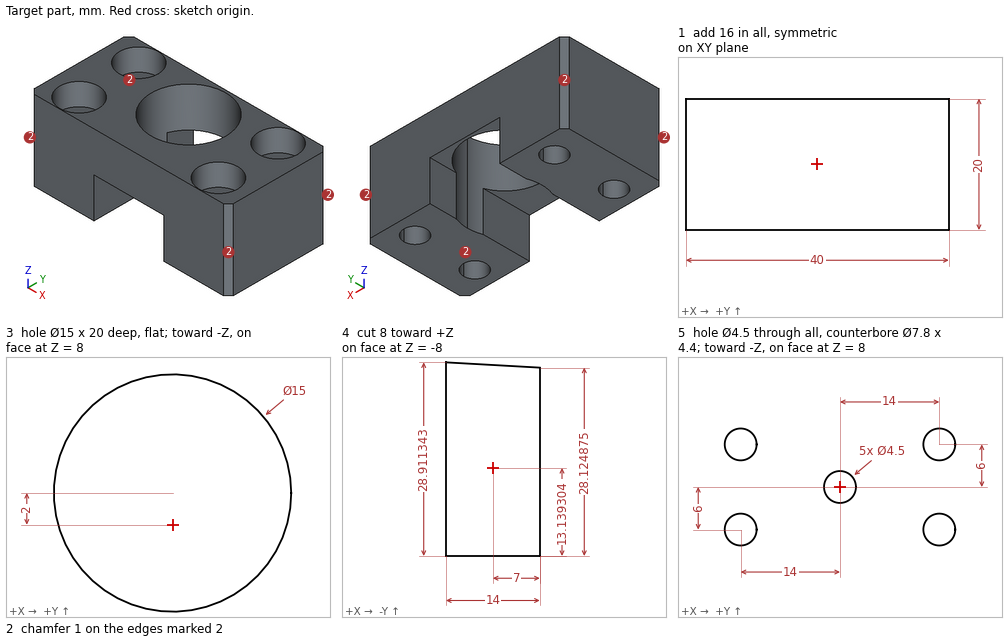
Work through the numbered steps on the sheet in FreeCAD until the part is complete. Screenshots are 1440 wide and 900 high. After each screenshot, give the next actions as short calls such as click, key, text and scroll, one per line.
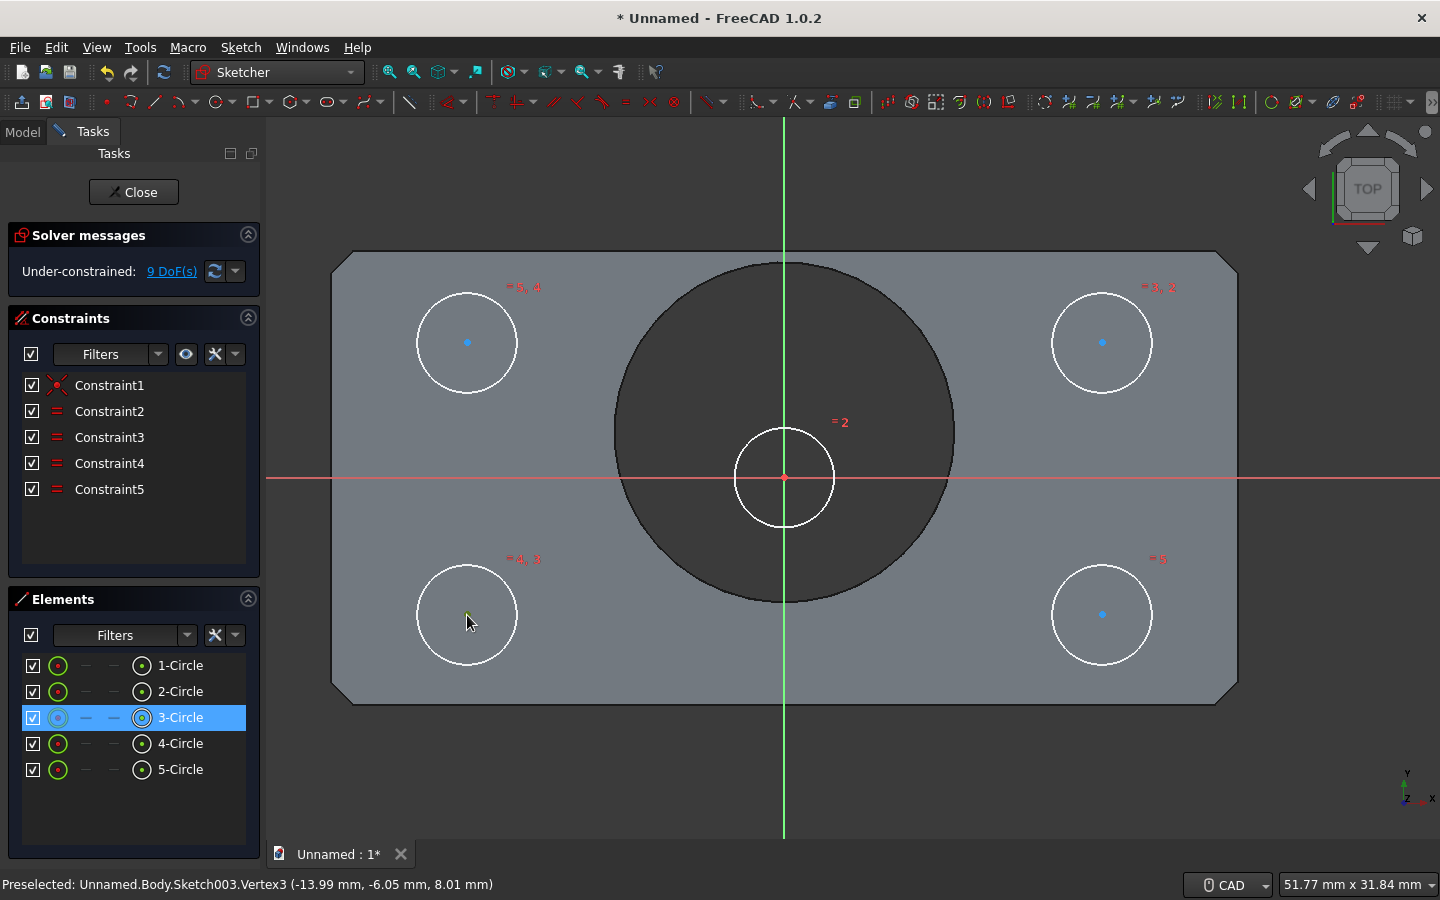
click(467, 343)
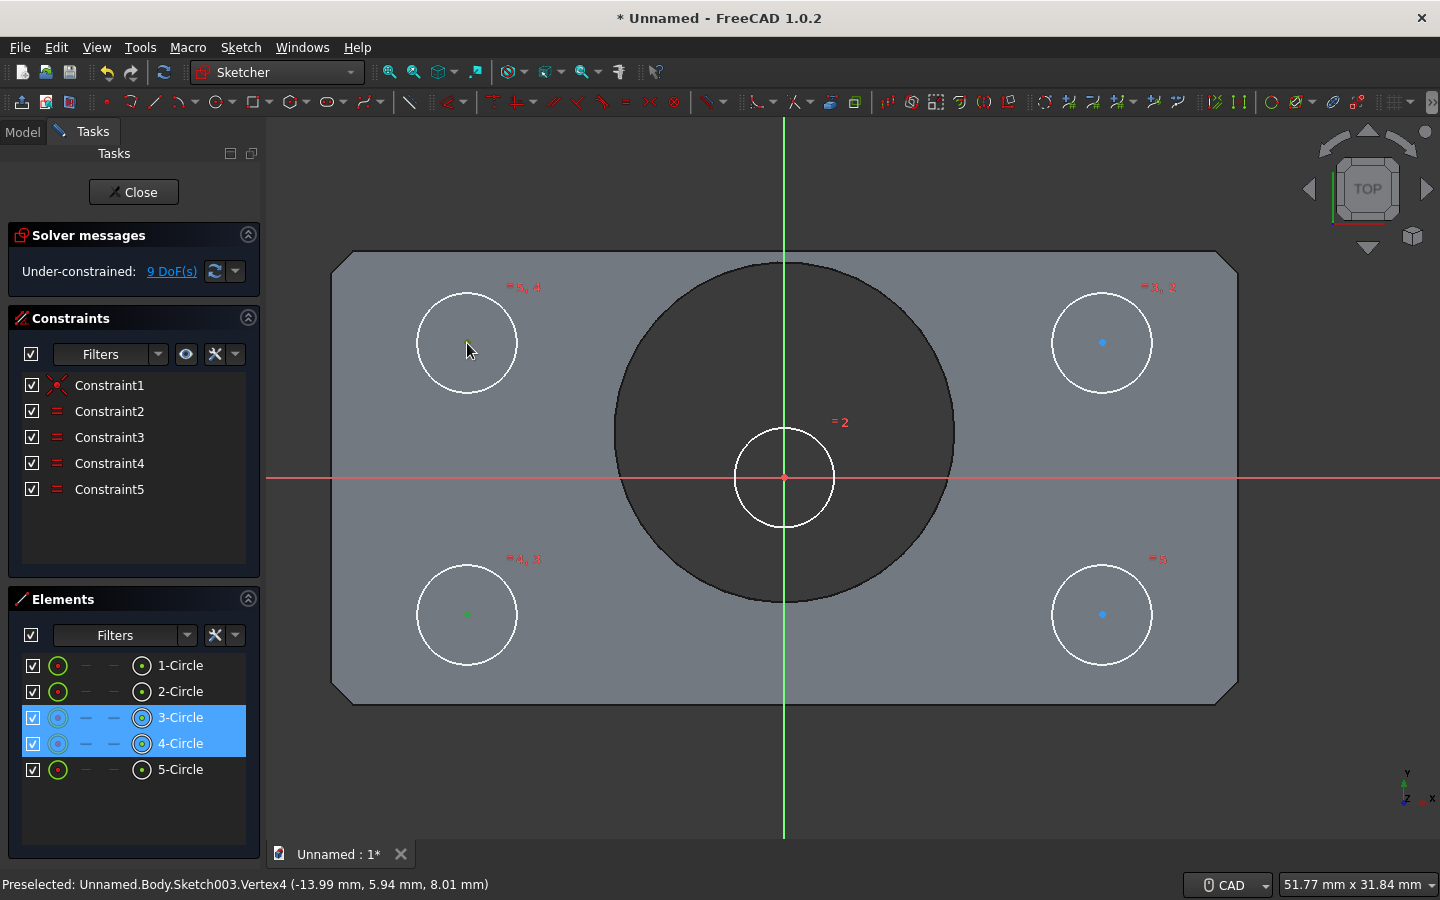
key(v)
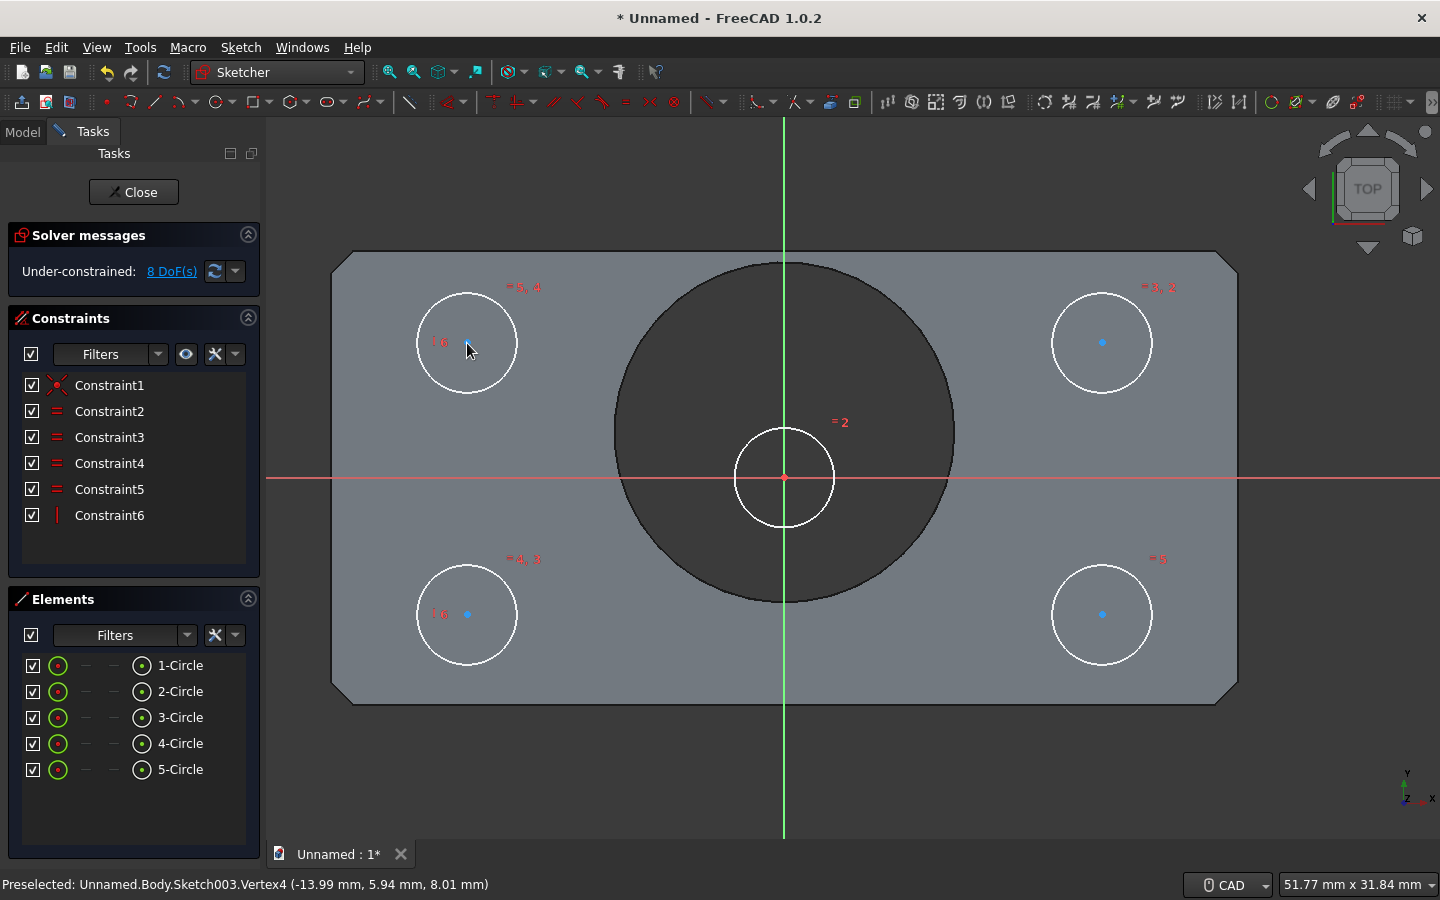
click(1102, 343)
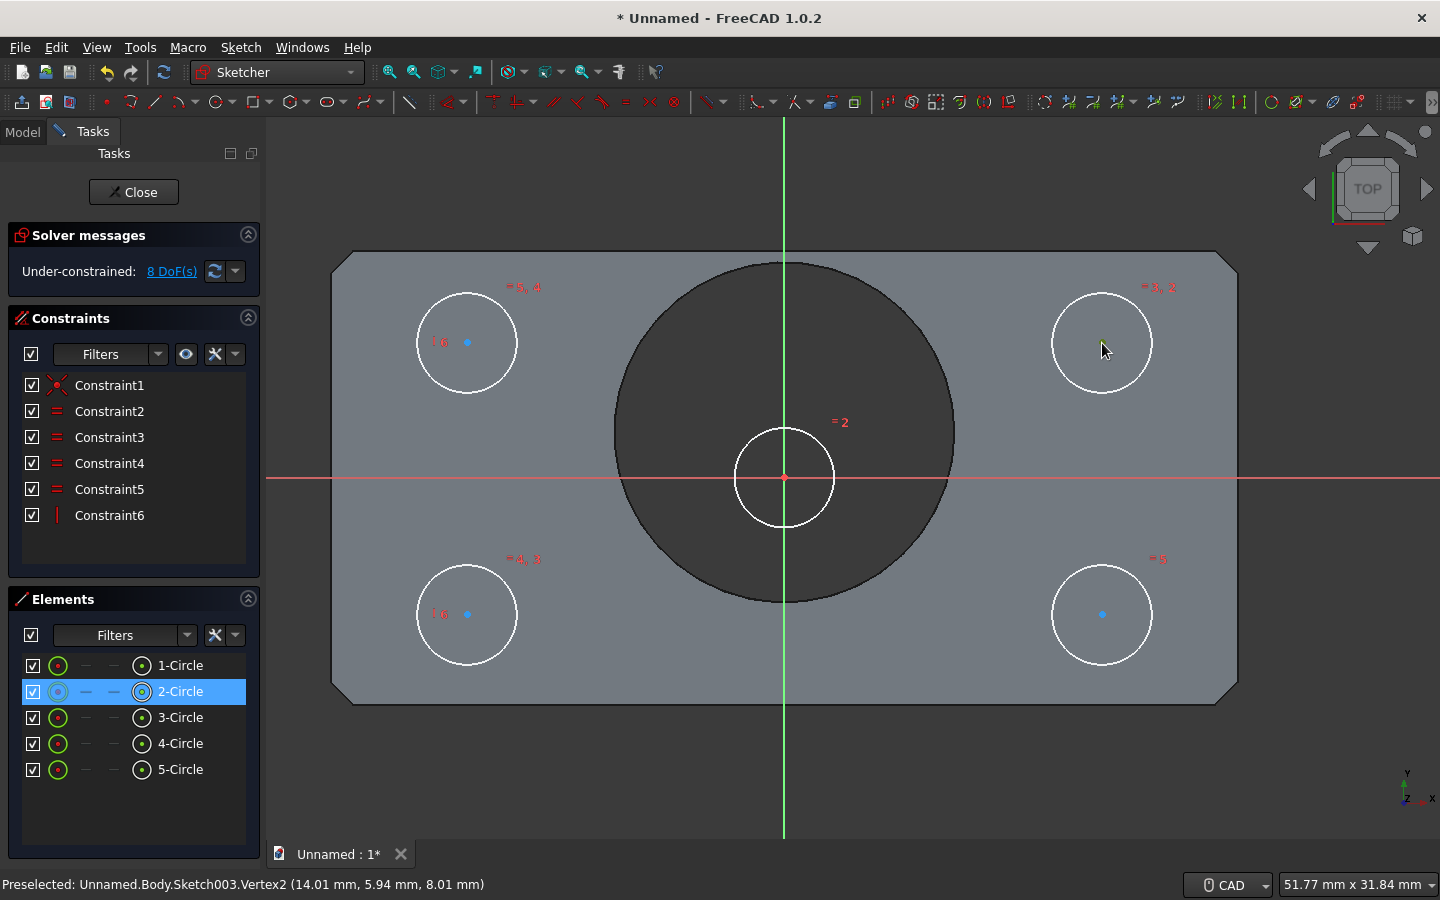
click(467, 343)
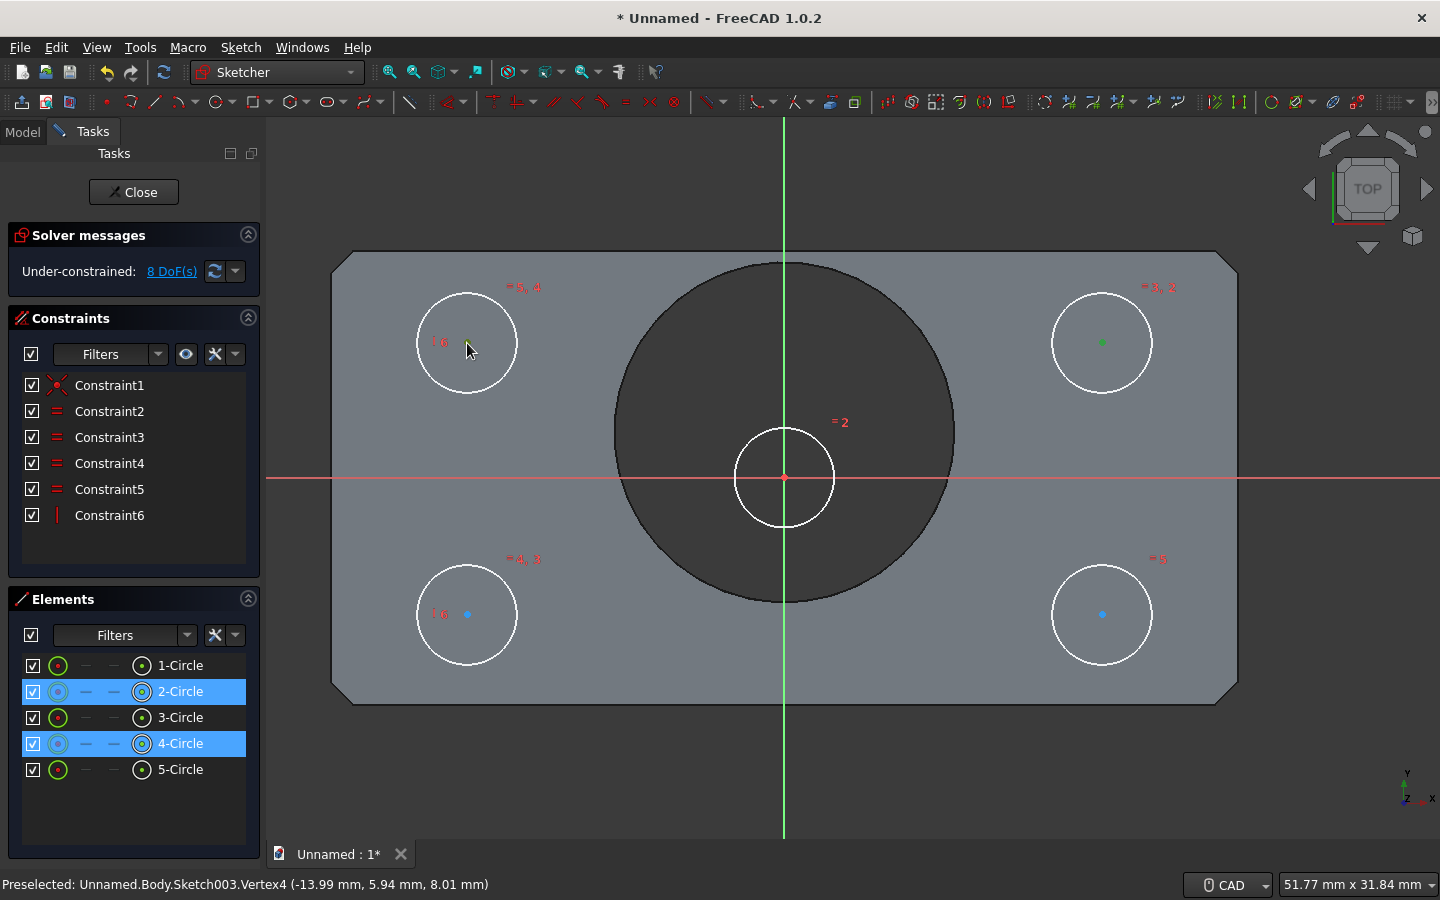
click(536, 102)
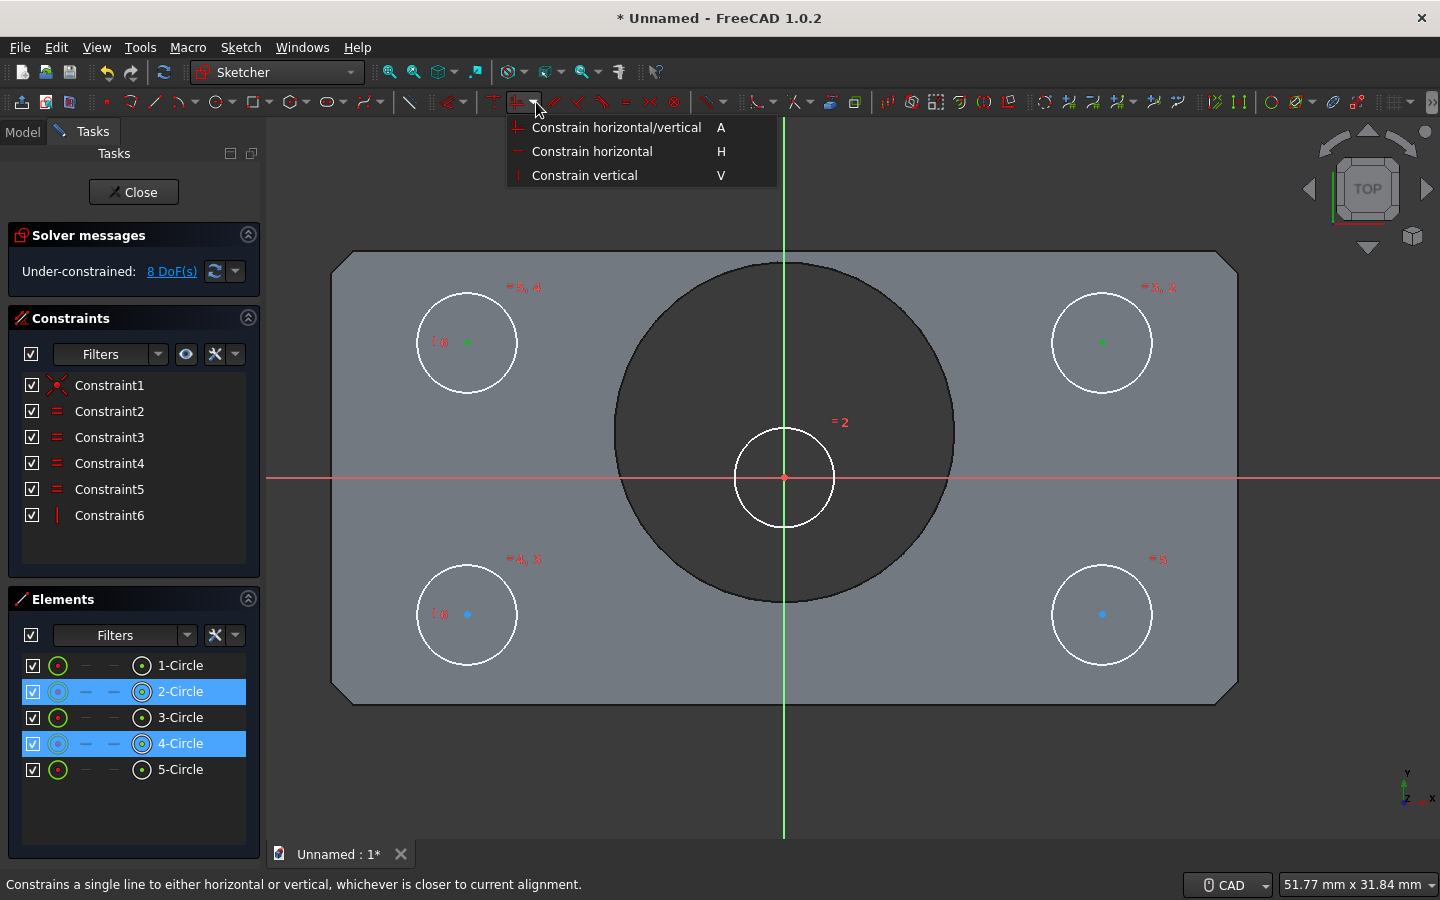
click(642, 151)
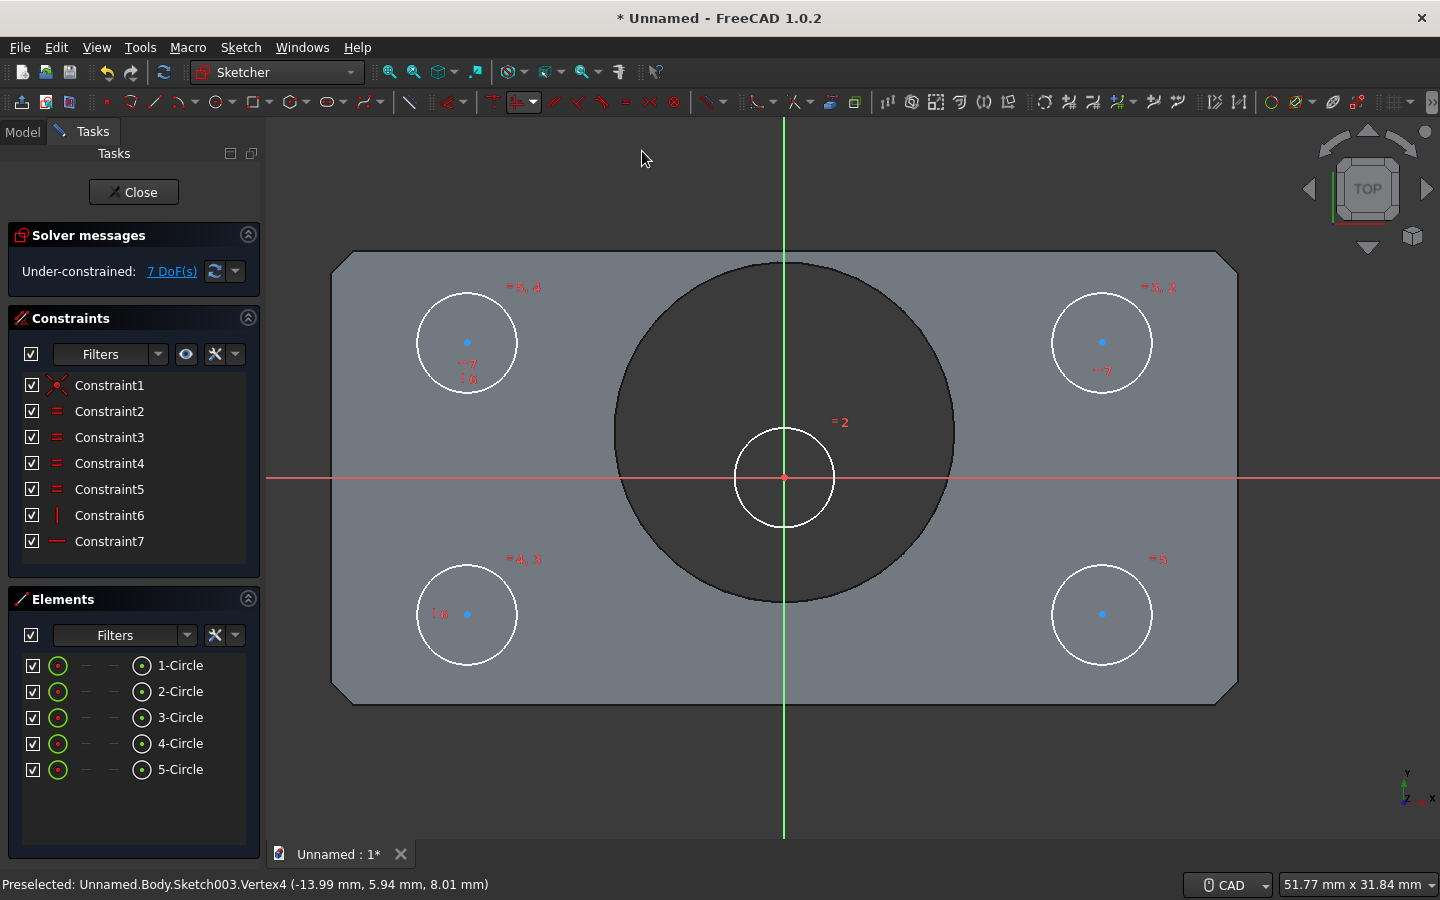
click(1102, 343)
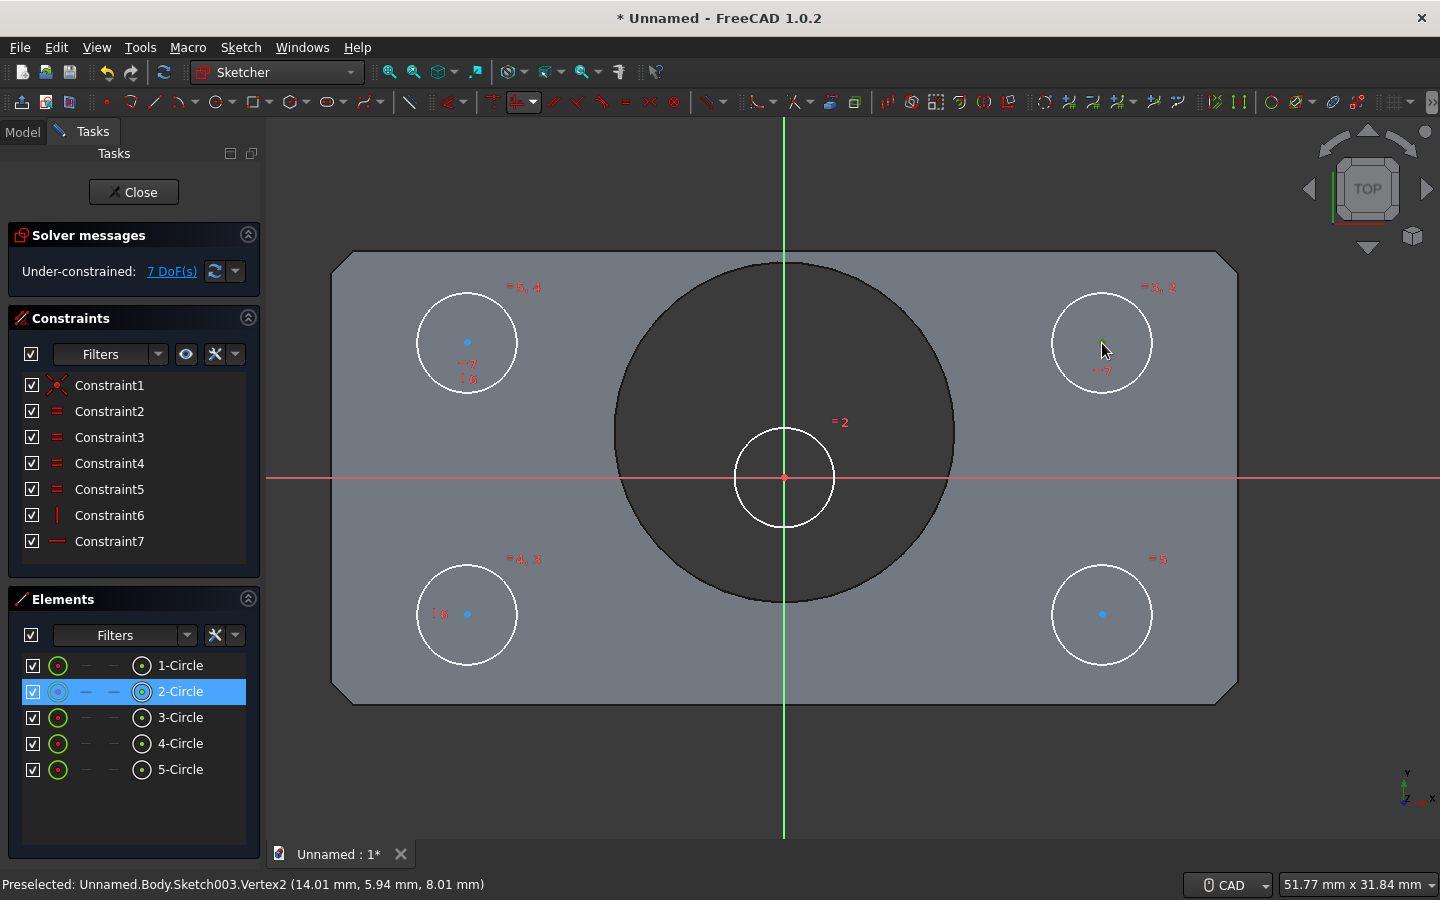
click(1102, 615)